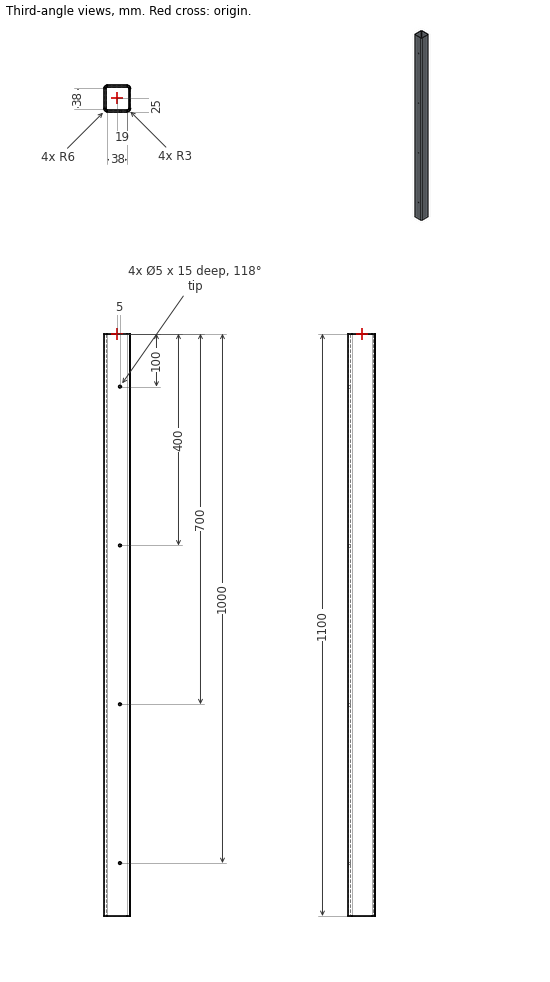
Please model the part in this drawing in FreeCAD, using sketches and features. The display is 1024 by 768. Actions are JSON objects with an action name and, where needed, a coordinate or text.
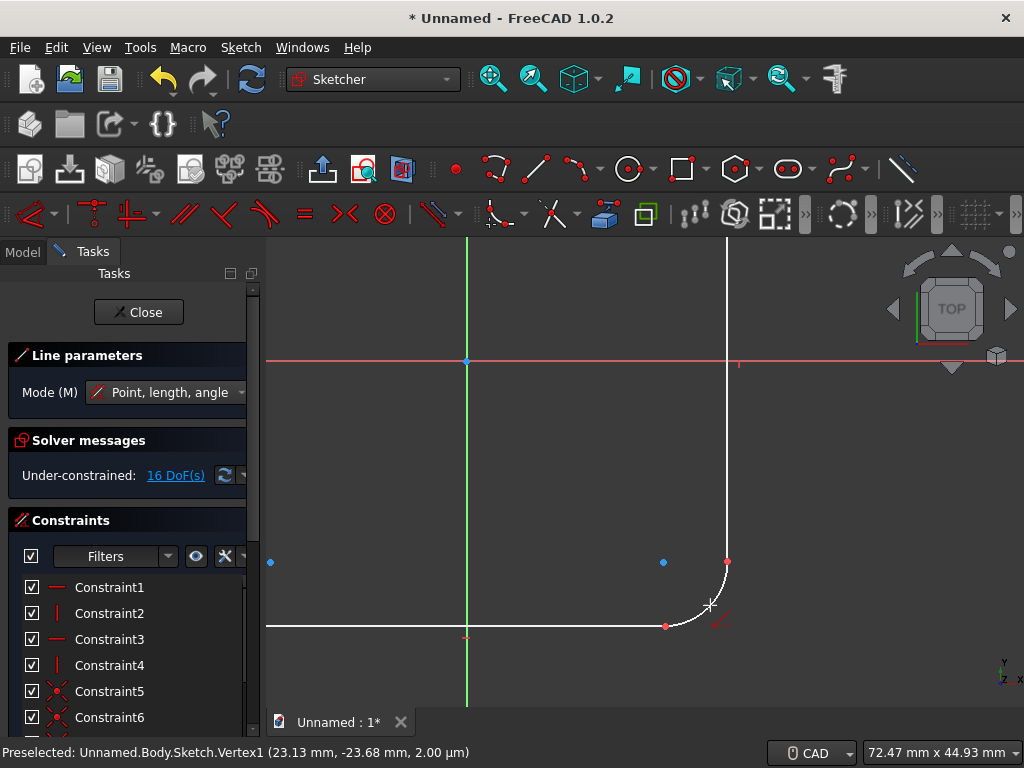
{"action": "scroll", "coordinate": [710, 607], "scroll_direction": "down", "scroll_amount": 3}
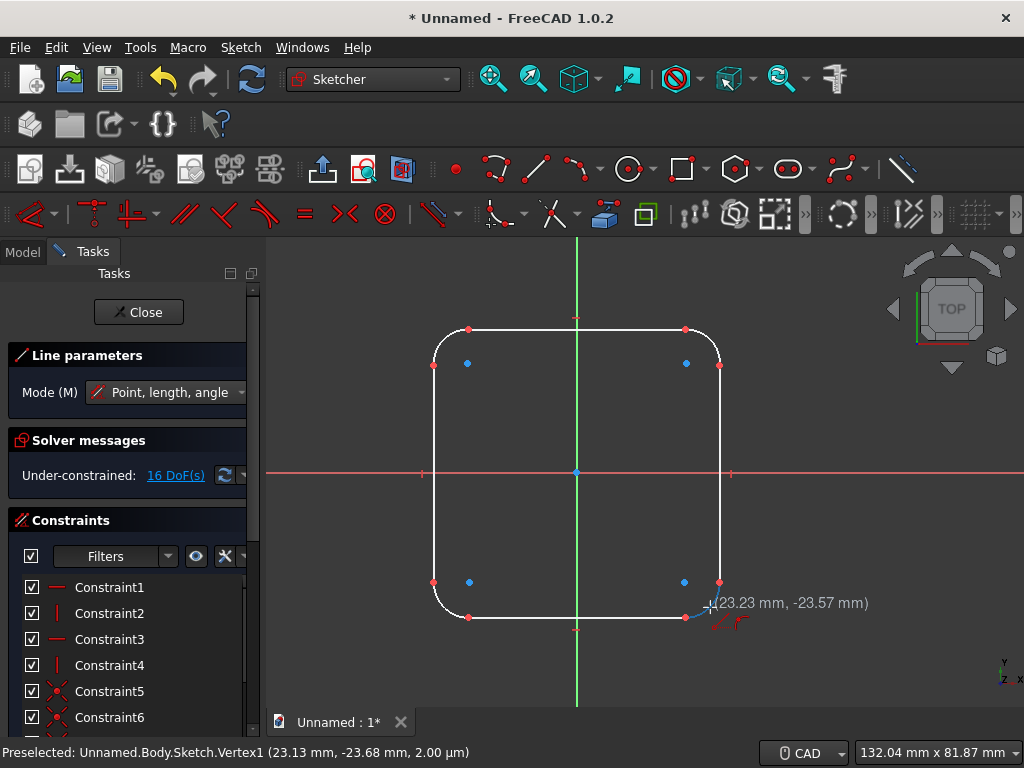
{"action": "left_click", "coordinate": [468, 599]}
{"action": "left_click", "coordinate": [686, 599]}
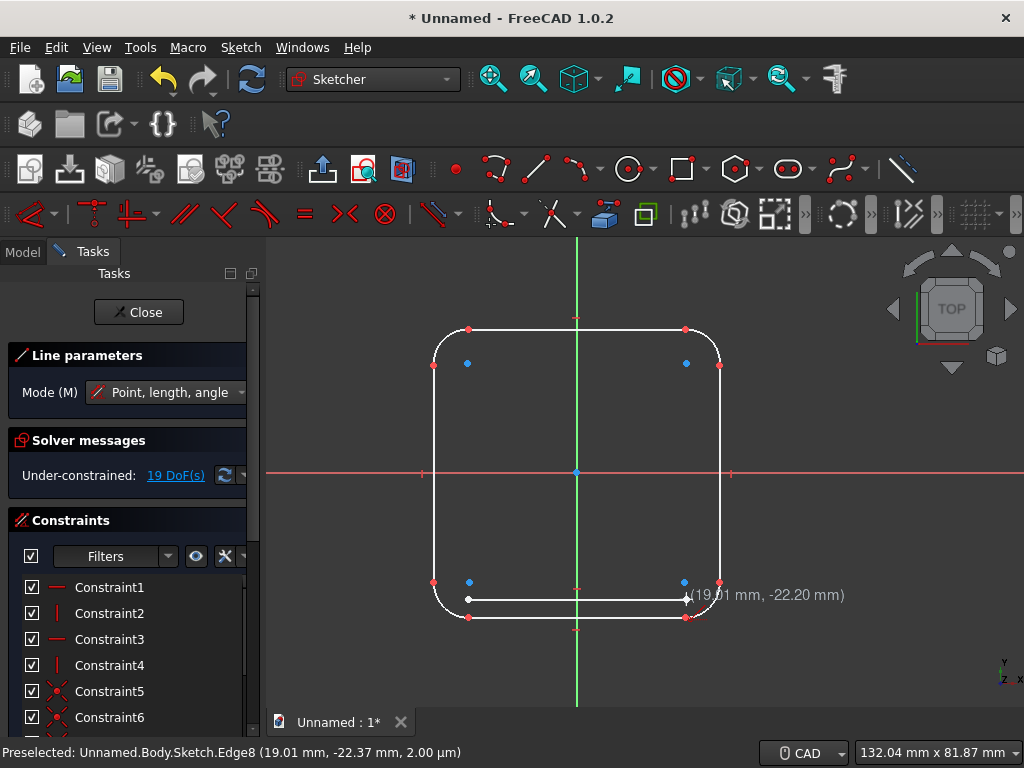
{"action": "left_click", "coordinate": [703, 582]}
{"action": "left_click", "coordinate": [703, 364]}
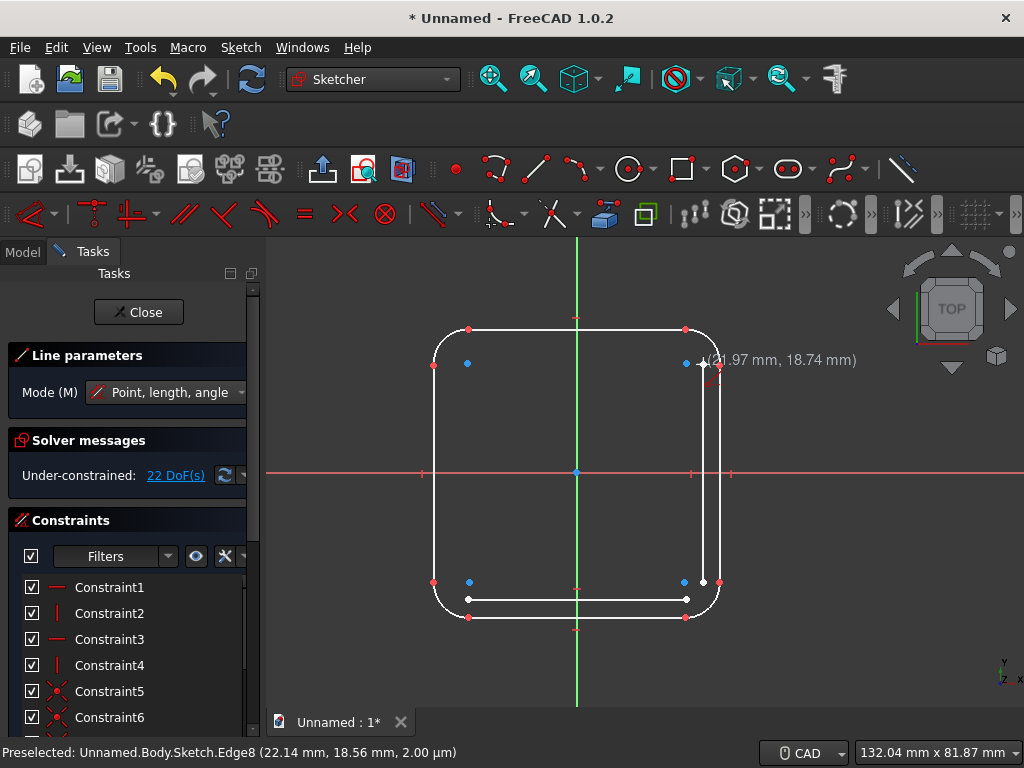
{"action": "left_click", "coordinate": [686, 346]}
{"action": "left_click", "coordinate": [468, 346]}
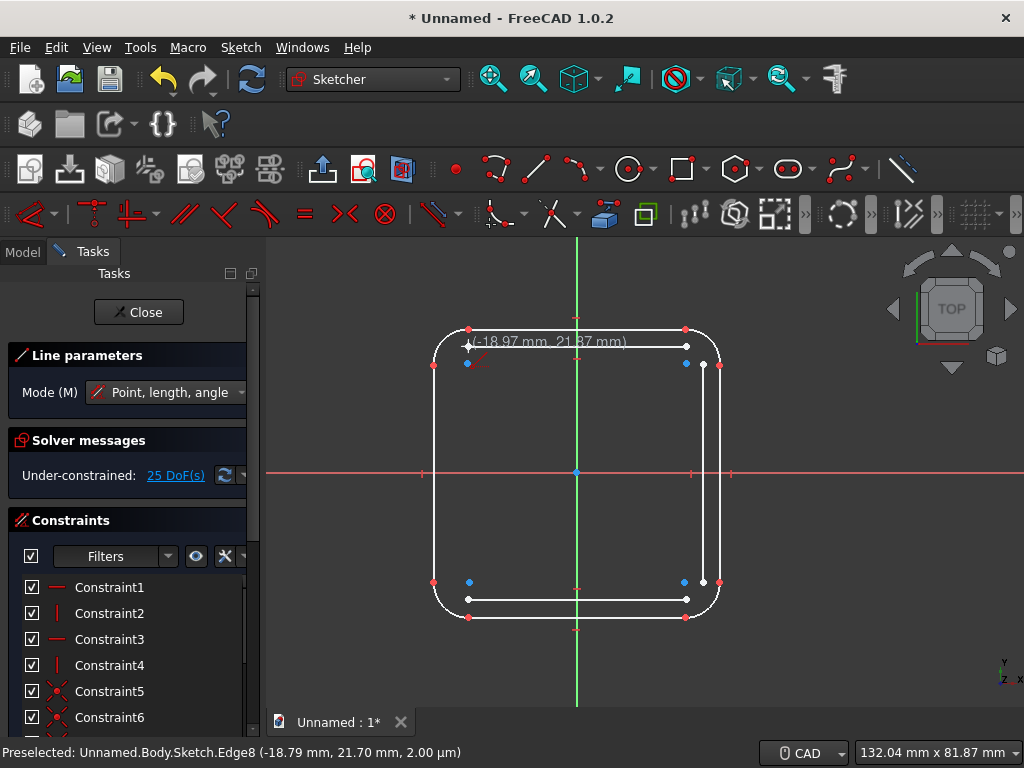
{"action": "left_click", "coordinate": [451, 364]}
{"action": "left_click", "coordinate": [451, 582]}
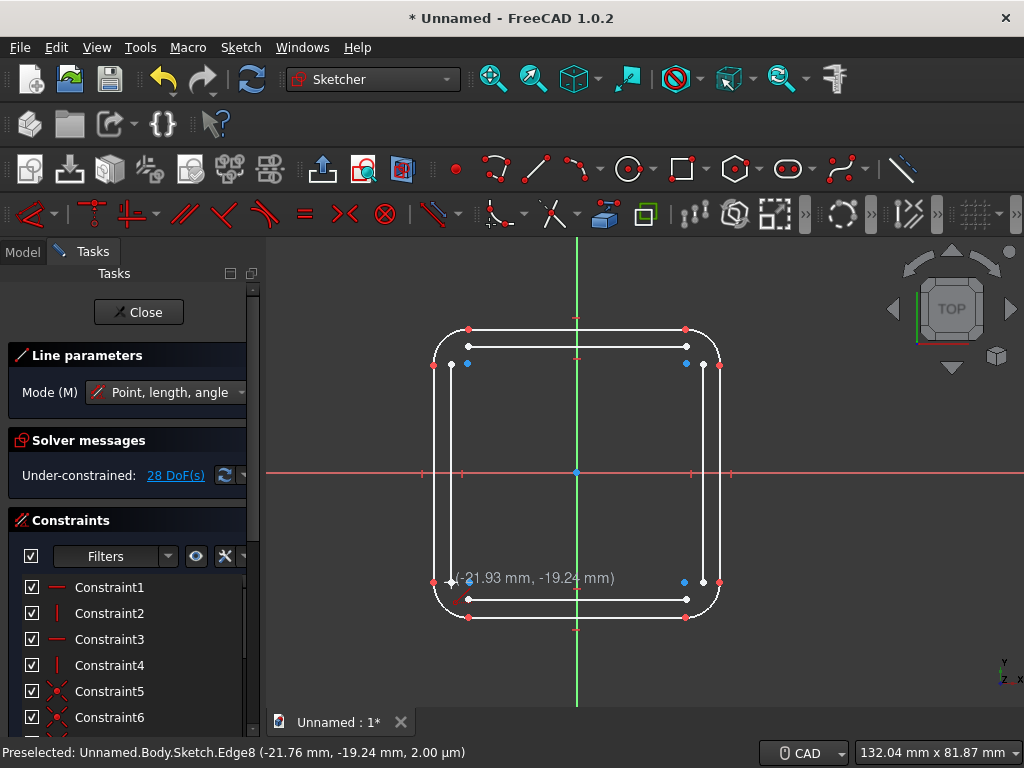
{"action": "key", "text": "g 3 a"}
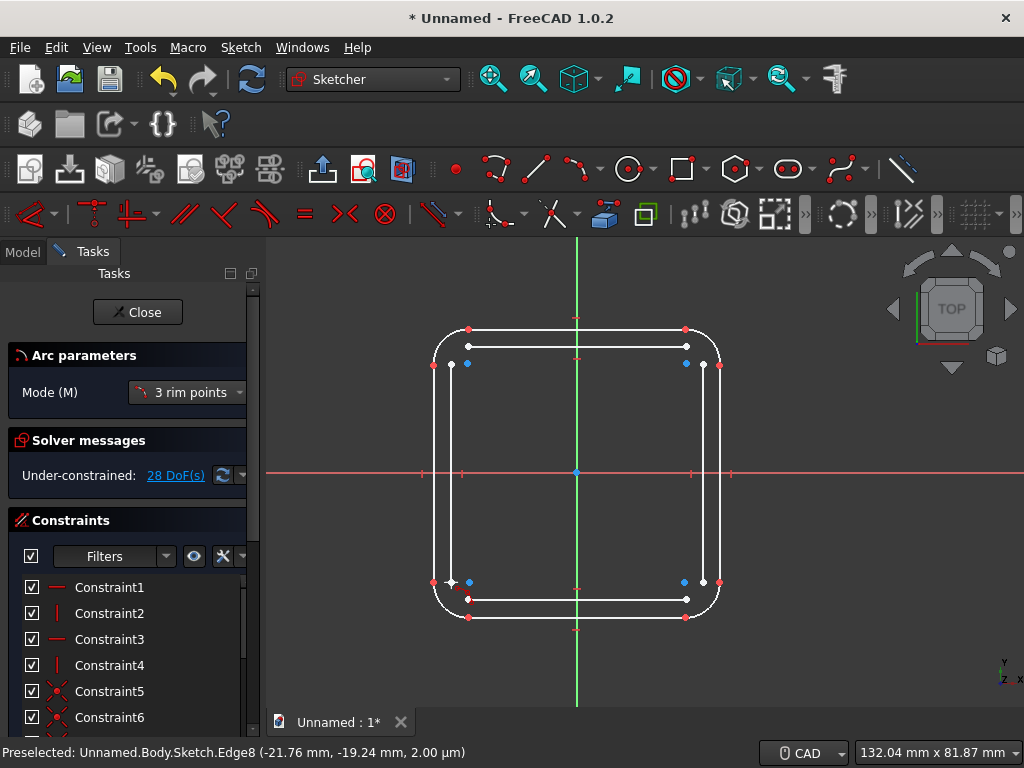
{"action": "left_click", "coordinate": [686, 600]}
{"action": "left_click", "coordinate": [703, 583]}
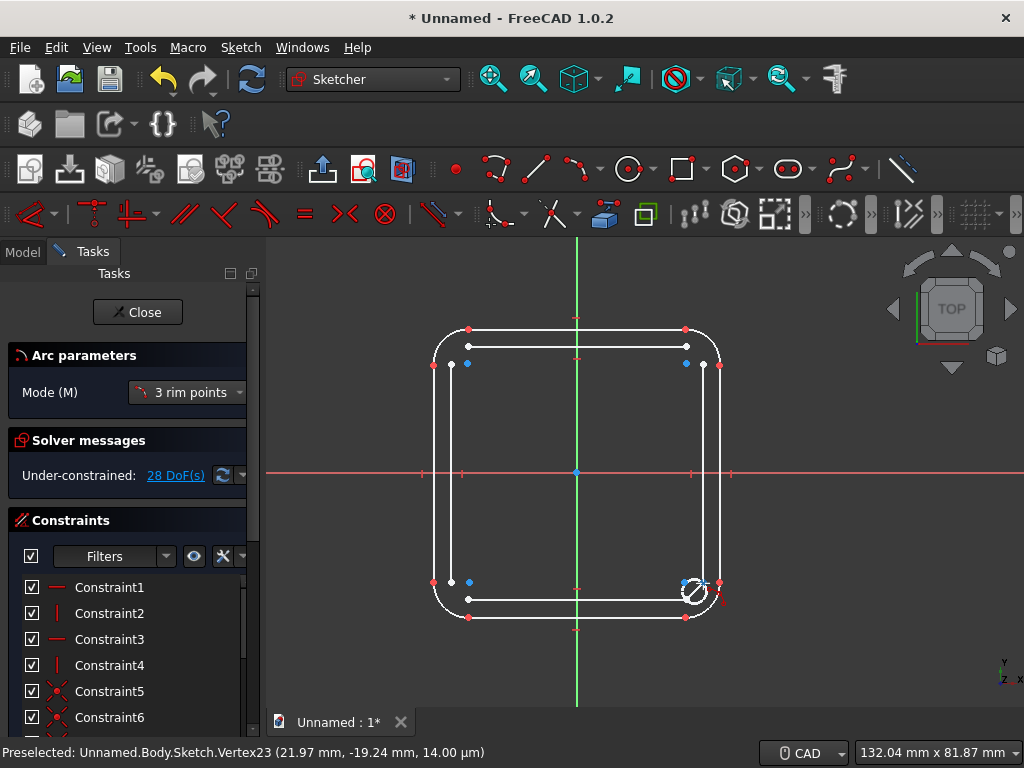
{"action": "scroll", "coordinate": [698, 594], "scroll_direction": "up", "scroll_amount": 6}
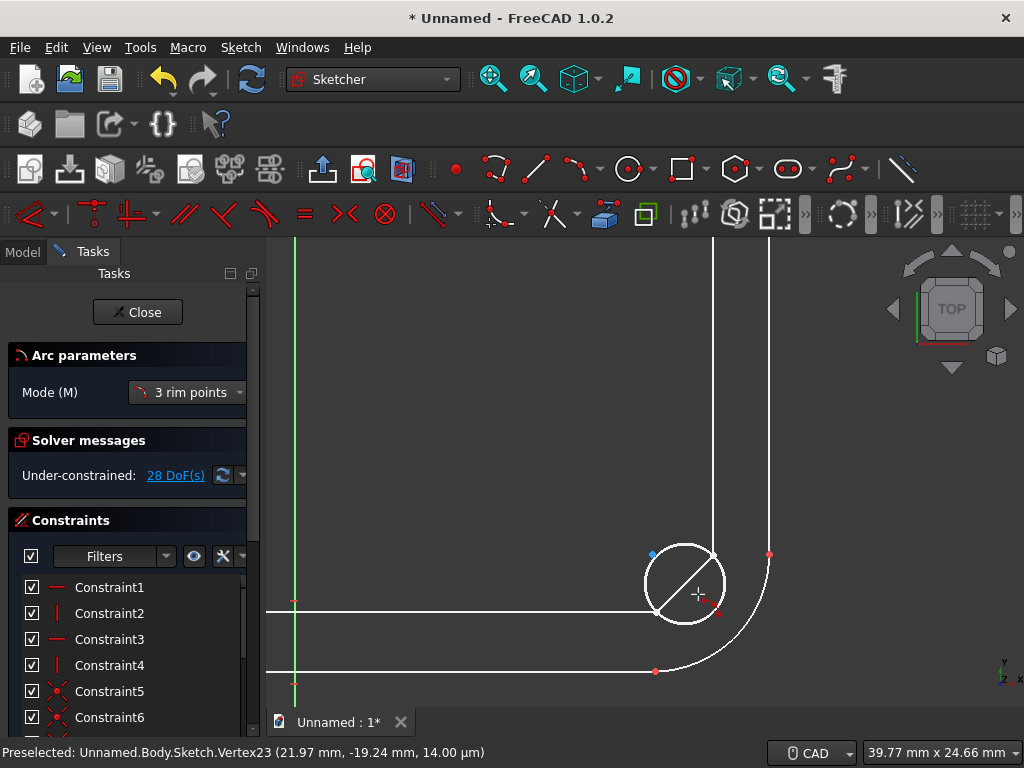
{"action": "left_click", "coordinate": [697, 592]}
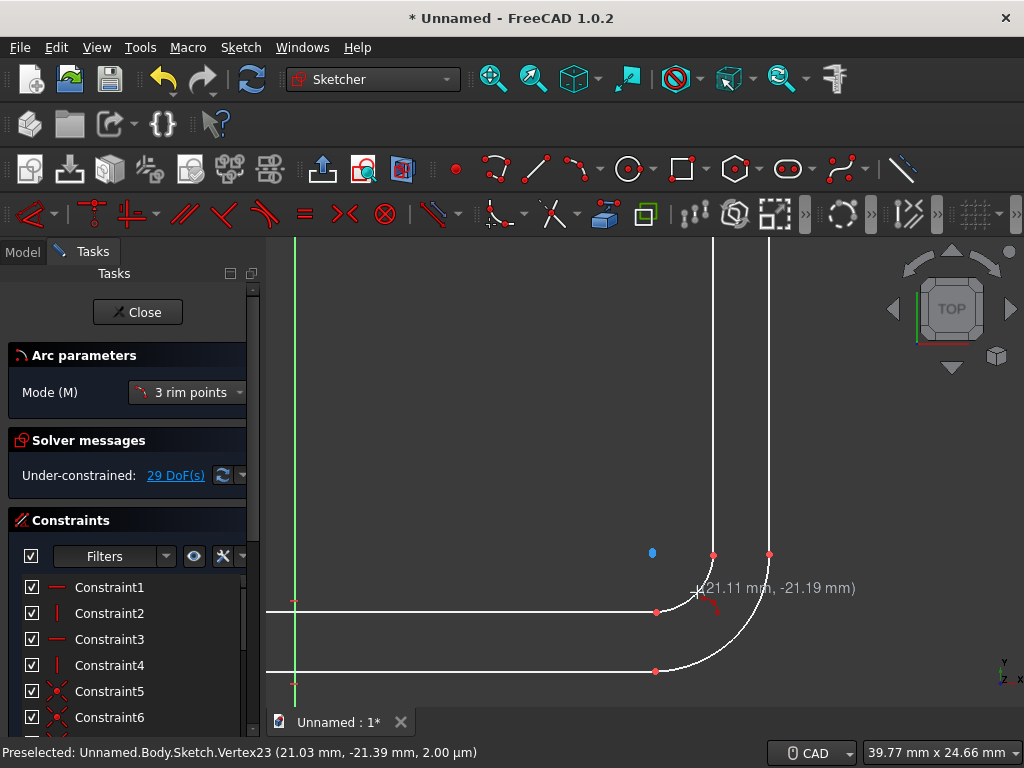
{"action": "scroll", "coordinate": [698, 594], "scroll_direction": "down", "scroll_amount": 6}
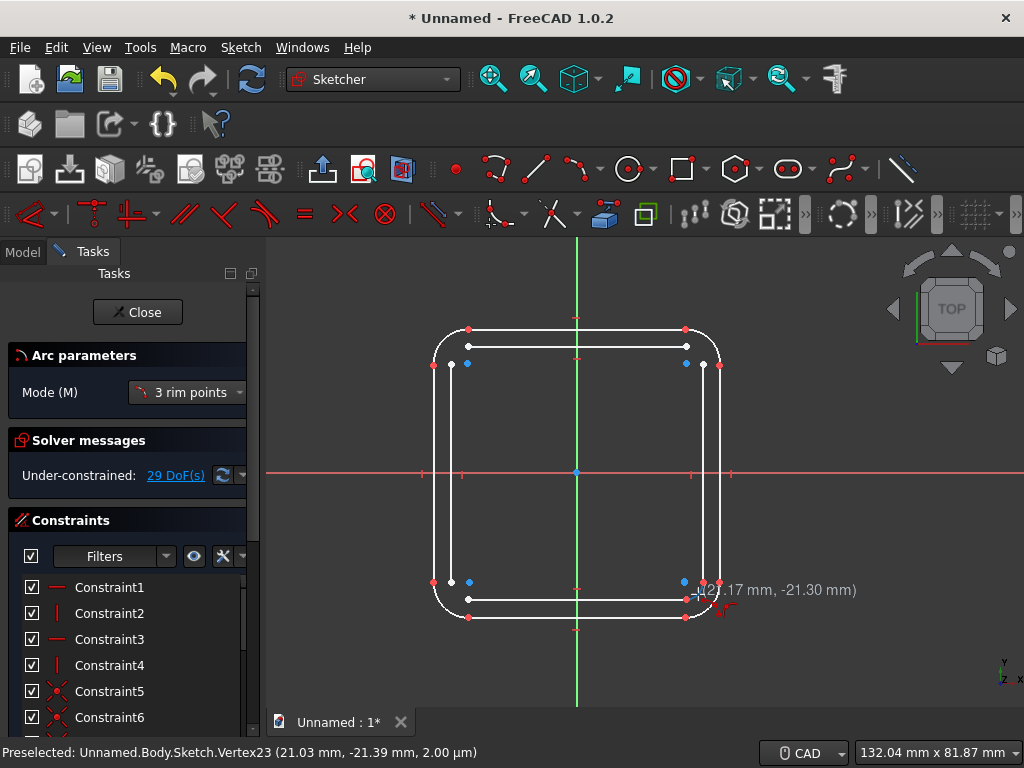
{"action": "left_click", "coordinate": [703, 365]}
{"action": "left_click", "coordinate": [686, 347]}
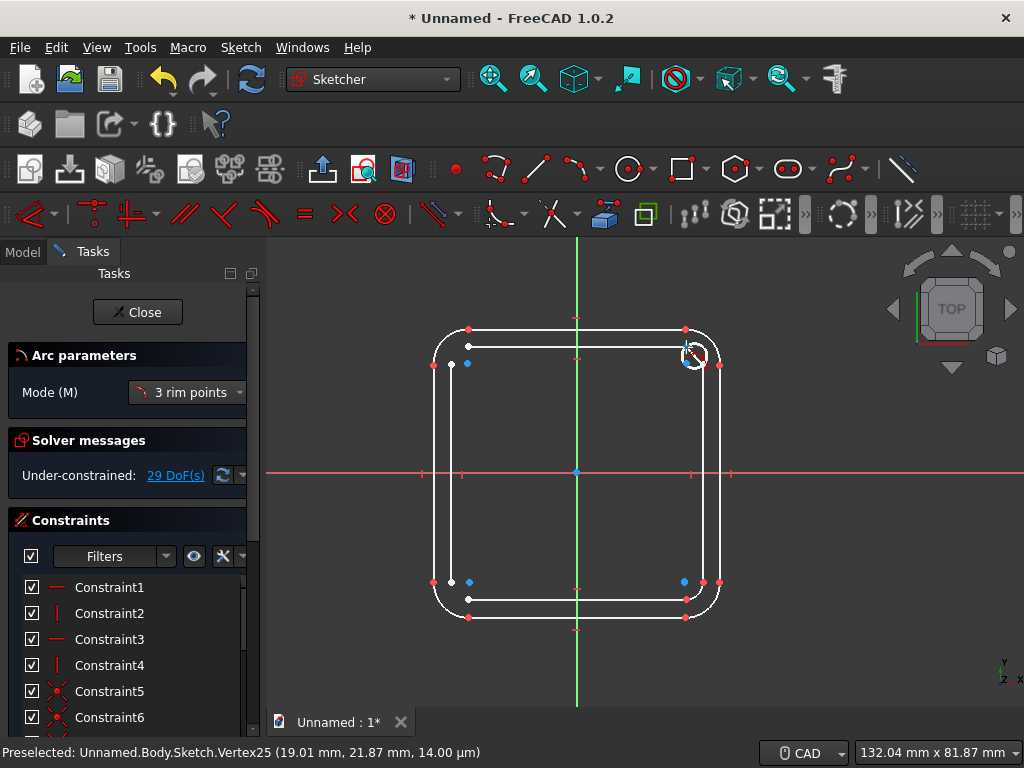
{"action": "scroll", "coordinate": [698, 351], "scroll_direction": "up", "scroll_amount": 6}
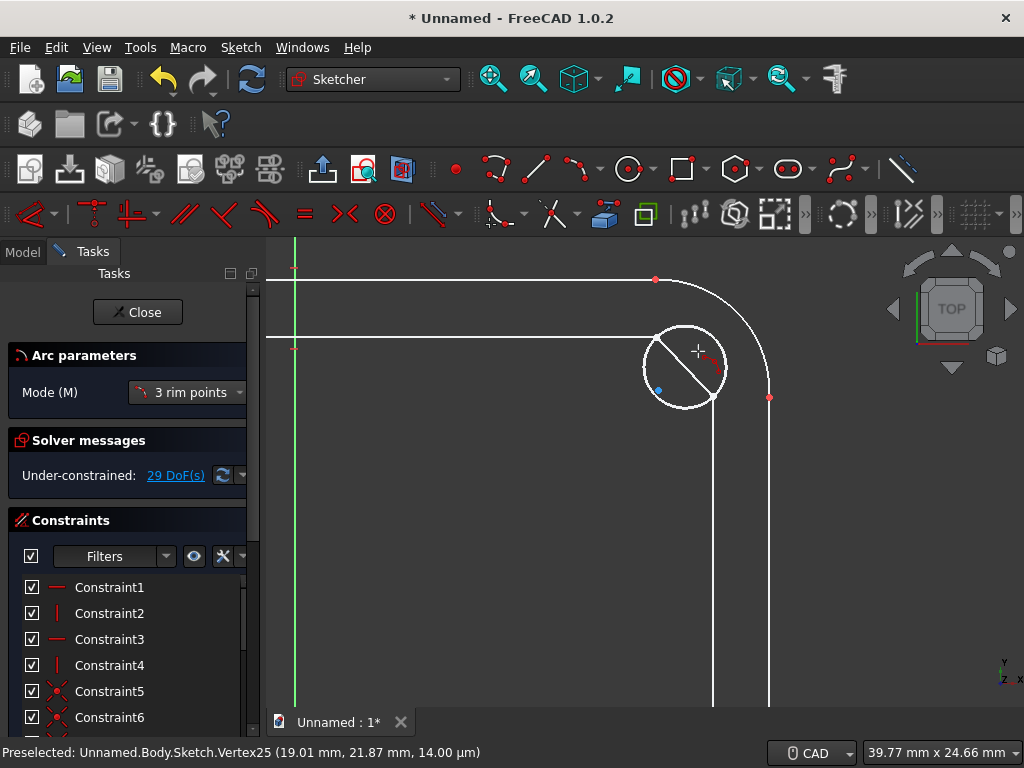
{"action": "left_click", "coordinate": [697, 352]}